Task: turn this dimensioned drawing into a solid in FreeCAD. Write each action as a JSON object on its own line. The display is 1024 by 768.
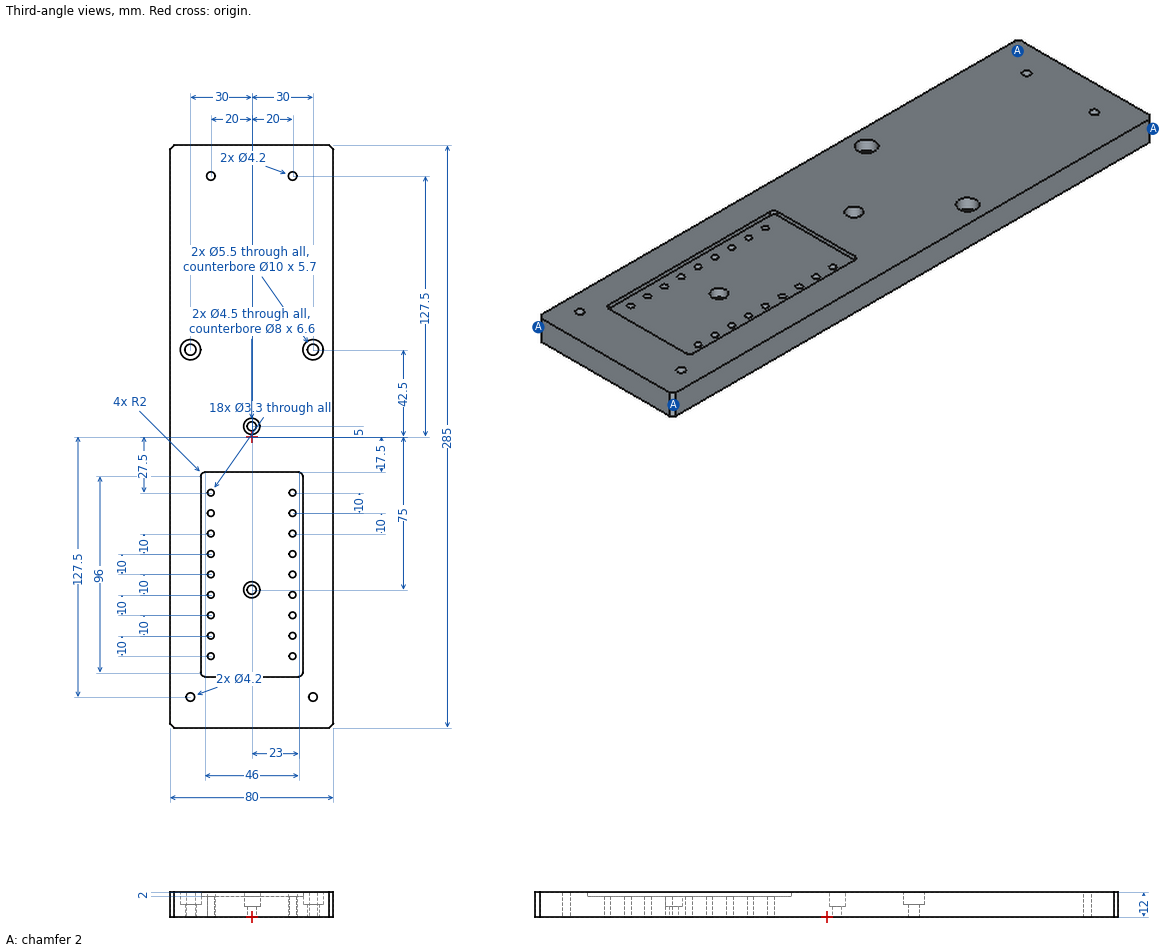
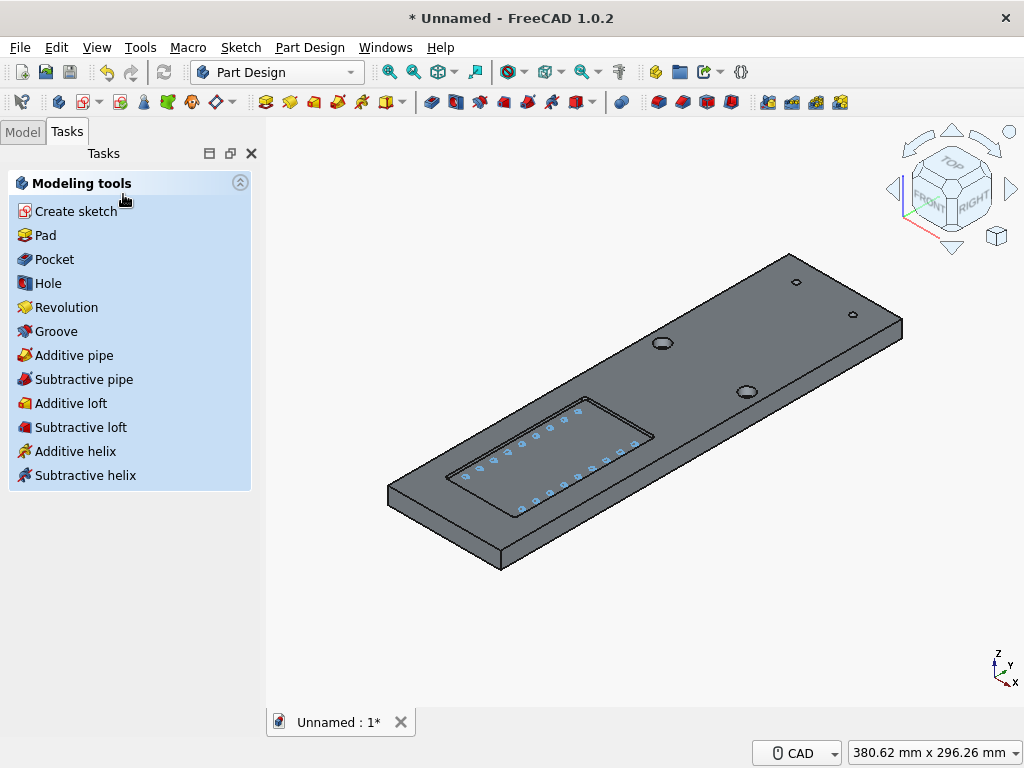
{"action": "left_click", "coordinate": [456, 102]}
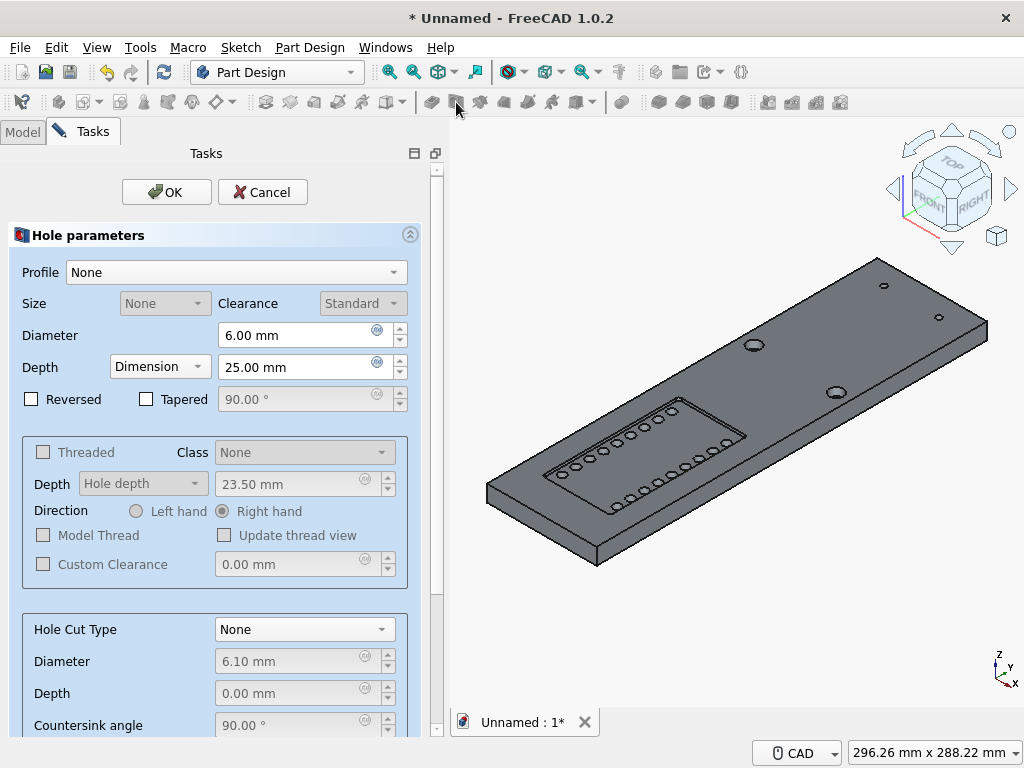
{"action": "triple_click", "coordinate": [305, 335]}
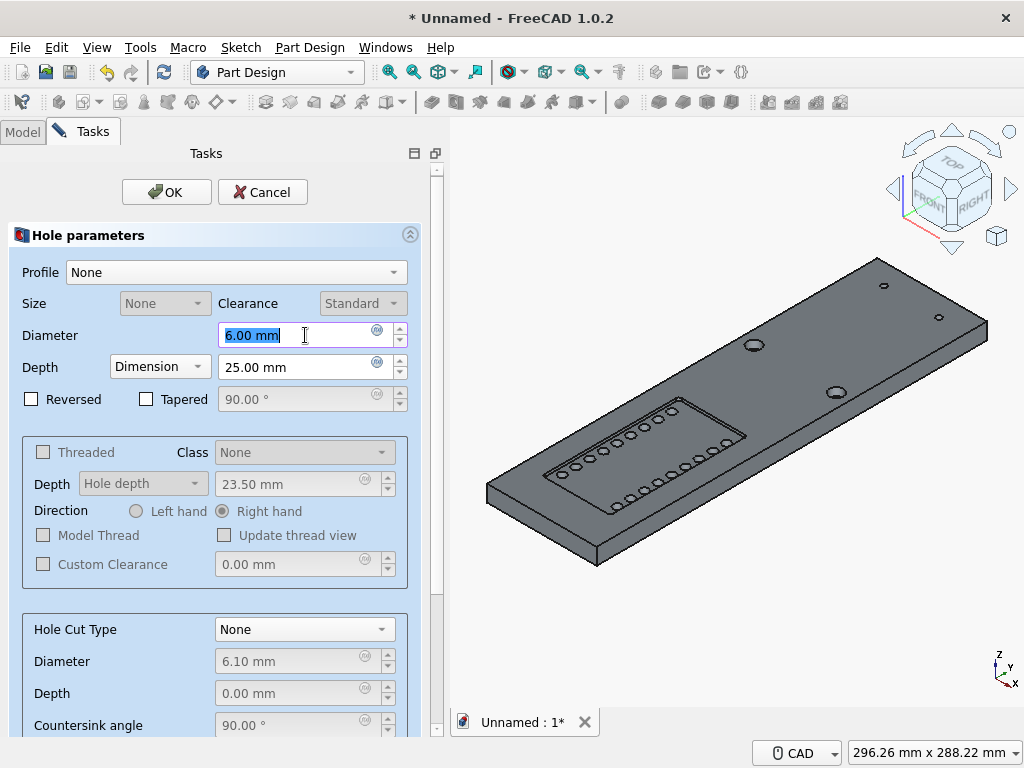
{"action": "type", "text": "3.3"}
{"action": "key", "text": "Tab"}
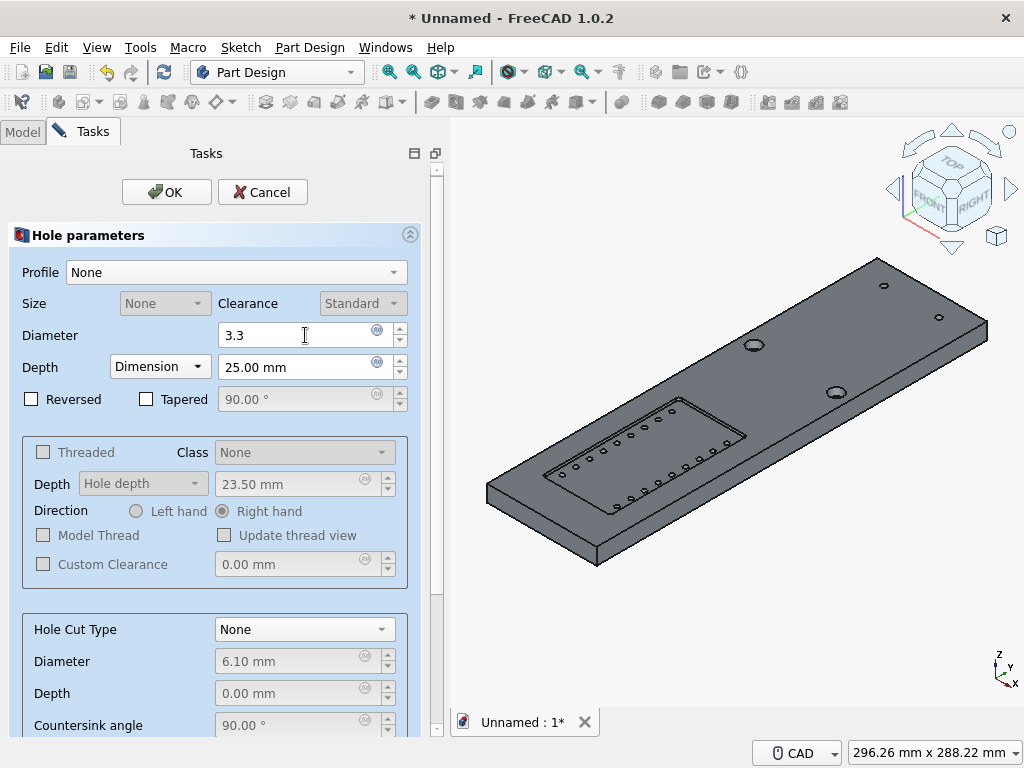
{"action": "left_click", "coordinate": [161, 366]}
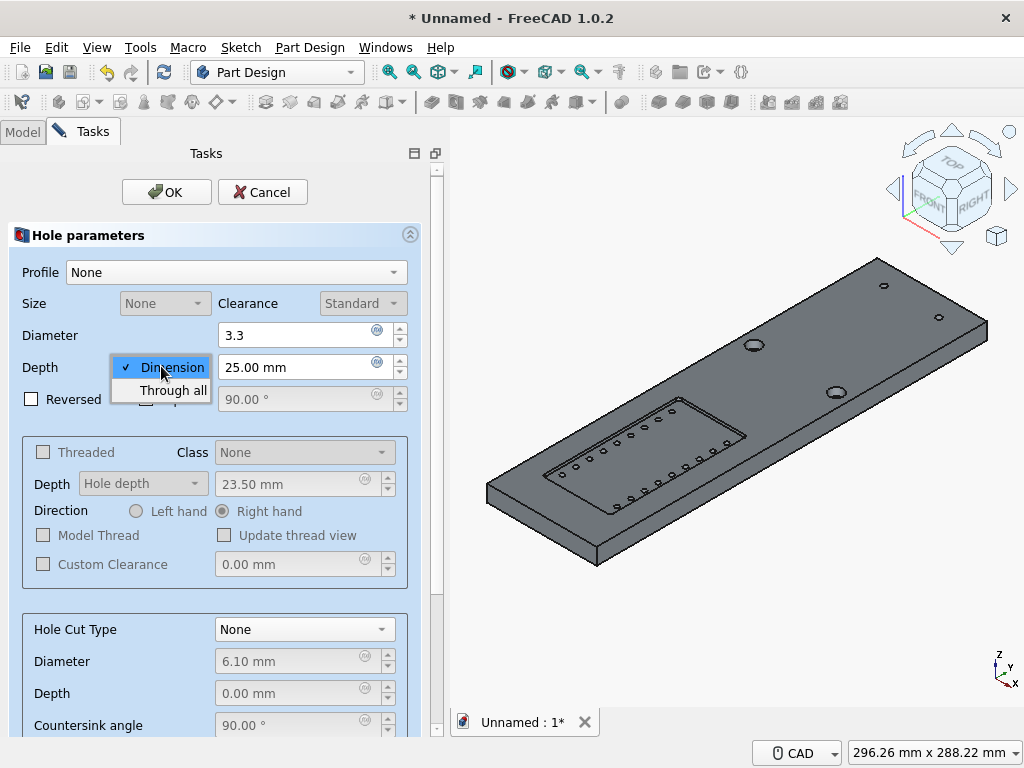
{"action": "left_click", "coordinate": [160, 390]}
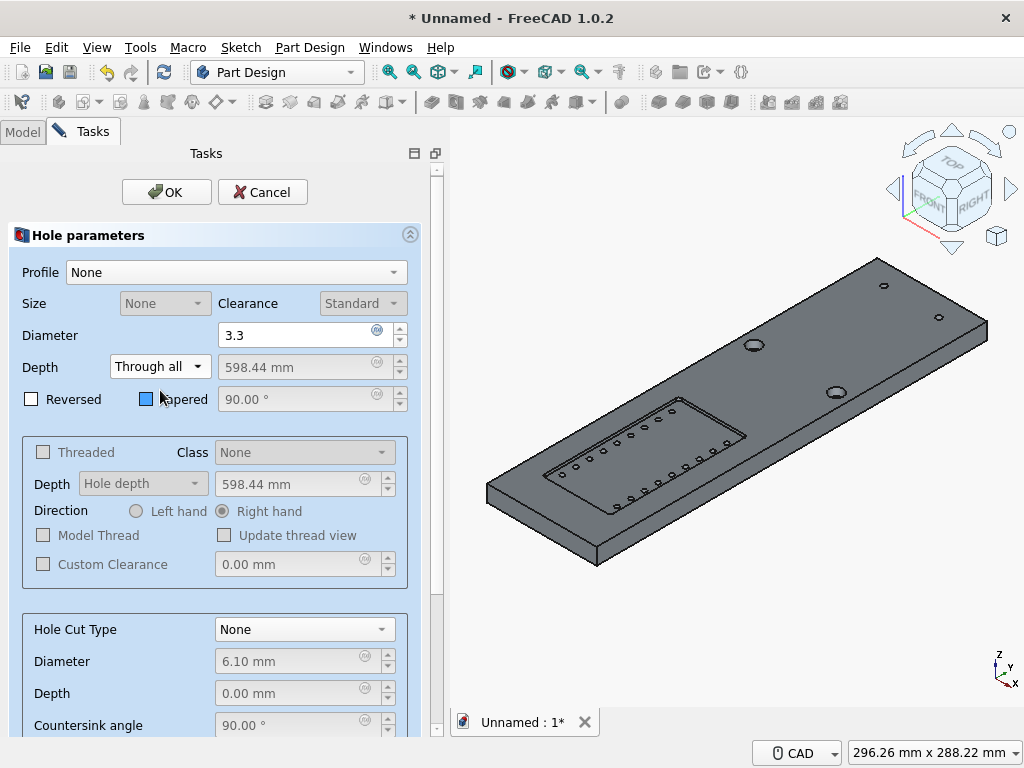
{"action": "left_click", "coordinate": [167, 192]}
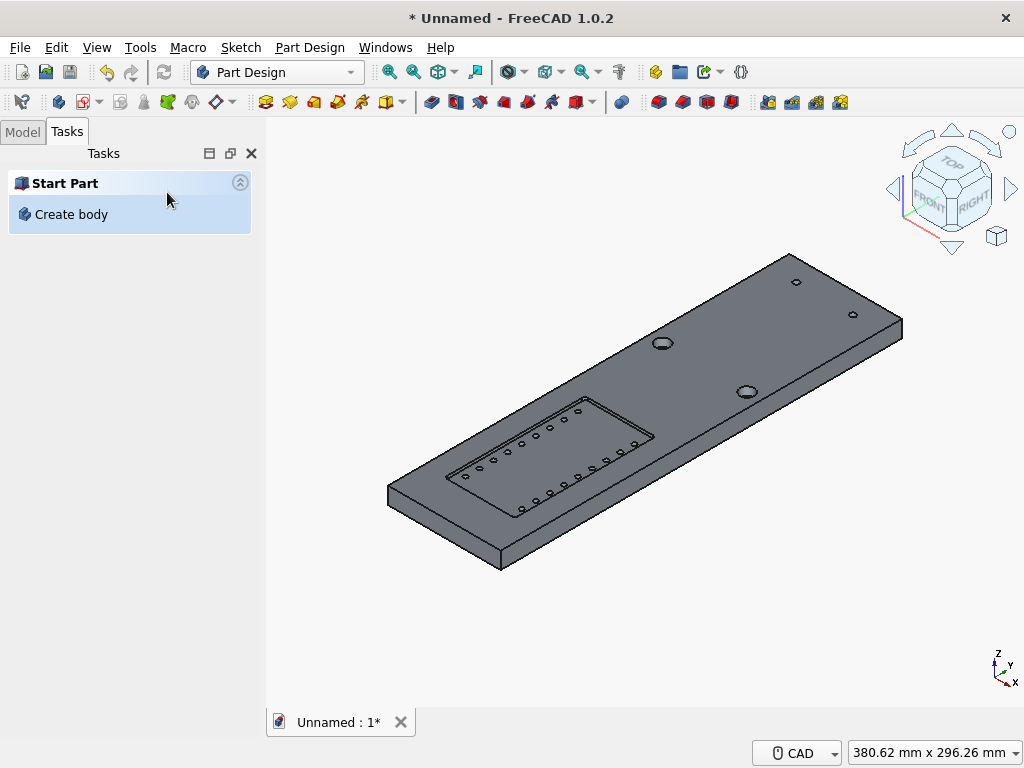
{"action": "left_click", "coordinate": [760, 335]}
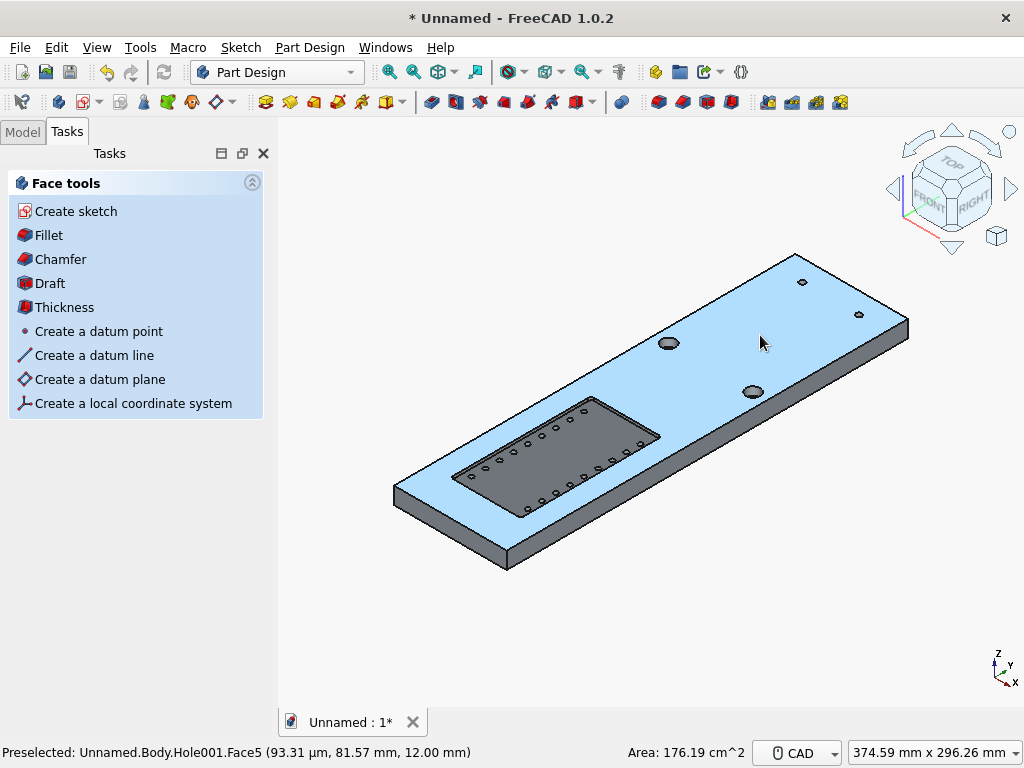
{"action": "left_click", "coordinate": [84, 102]}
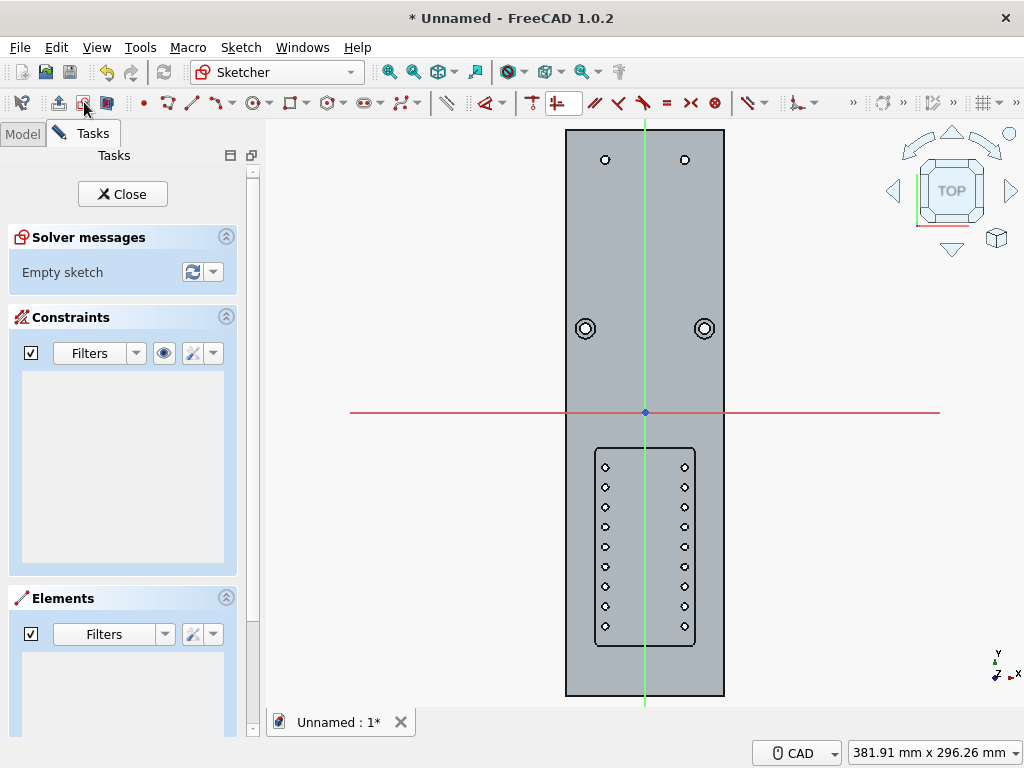
{"action": "scroll", "coordinate": [294, 147], "scroll_direction": "down", "scroll_amount": 1}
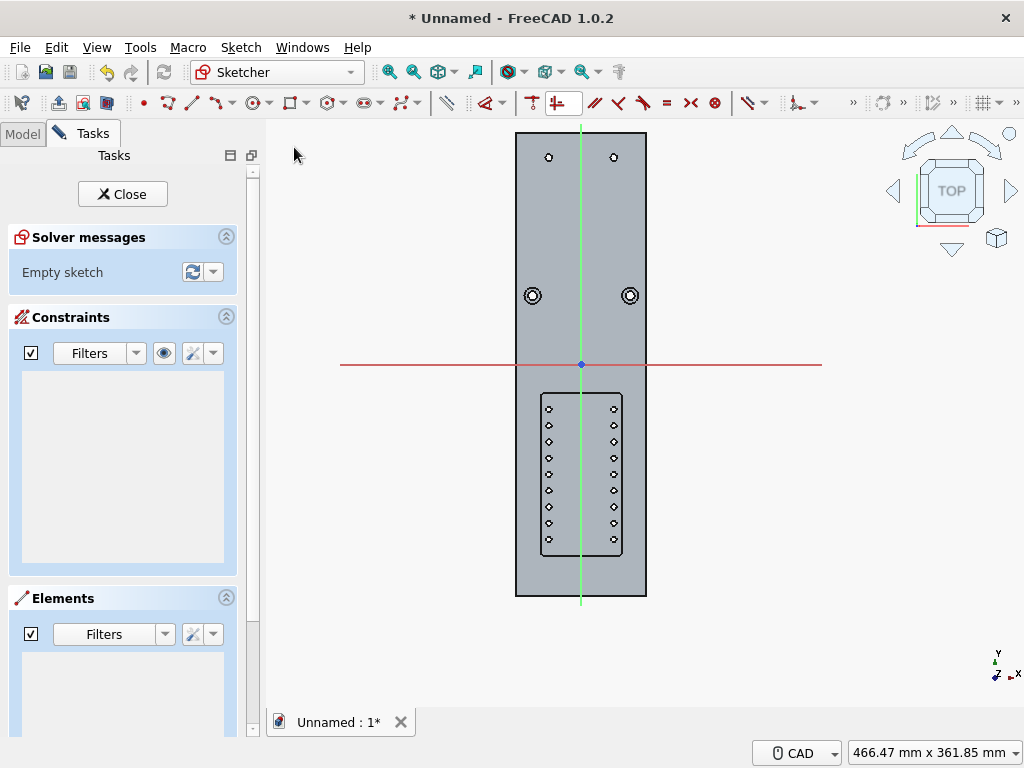
{"action": "scroll", "coordinate": [587, 540], "scroll_direction": "up", "scroll_amount": 3}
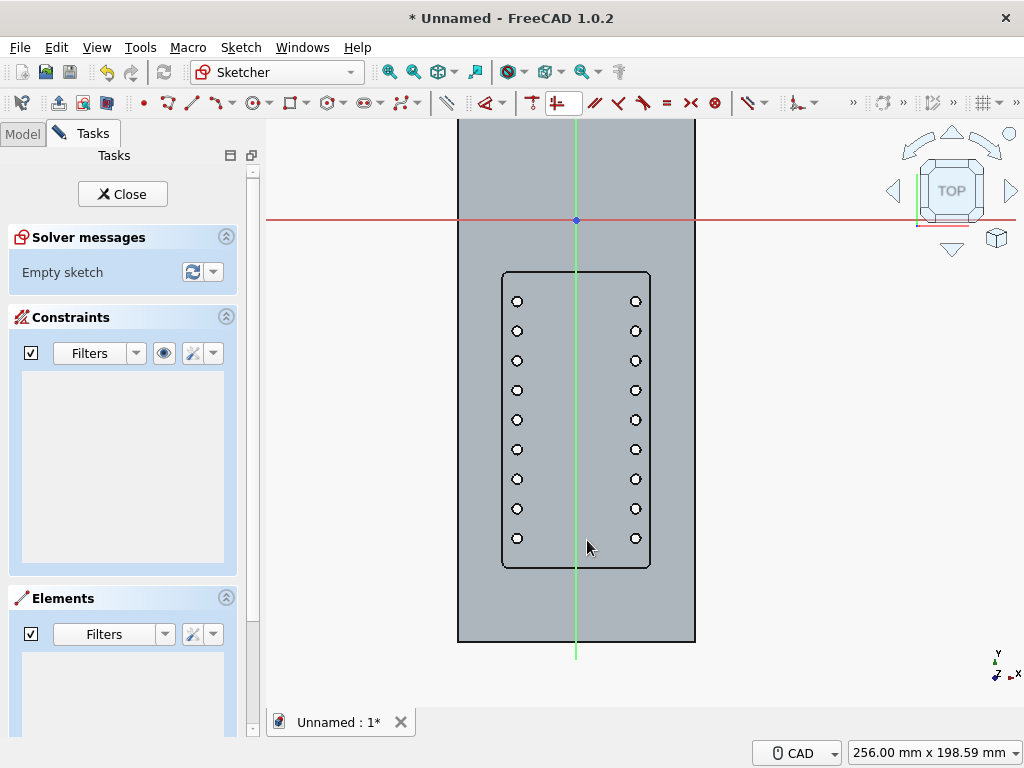
{"action": "left_click", "coordinate": [254, 104]}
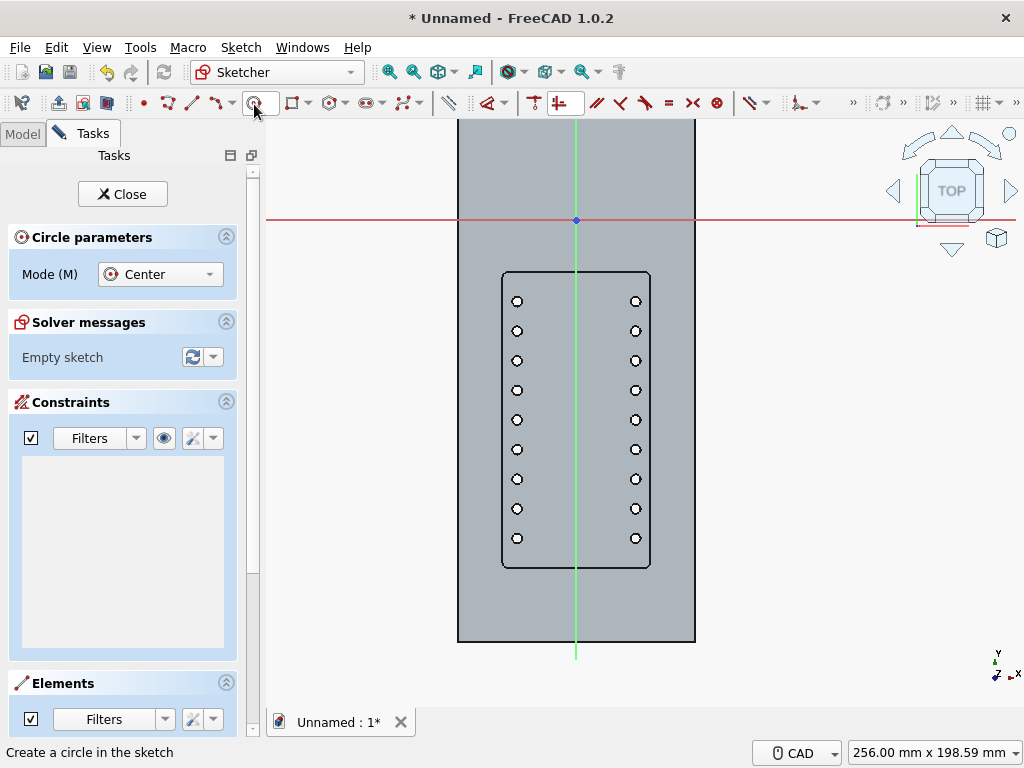
{"action": "scroll", "coordinate": [488, 598], "scroll_direction": "up", "scroll_amount": 7}